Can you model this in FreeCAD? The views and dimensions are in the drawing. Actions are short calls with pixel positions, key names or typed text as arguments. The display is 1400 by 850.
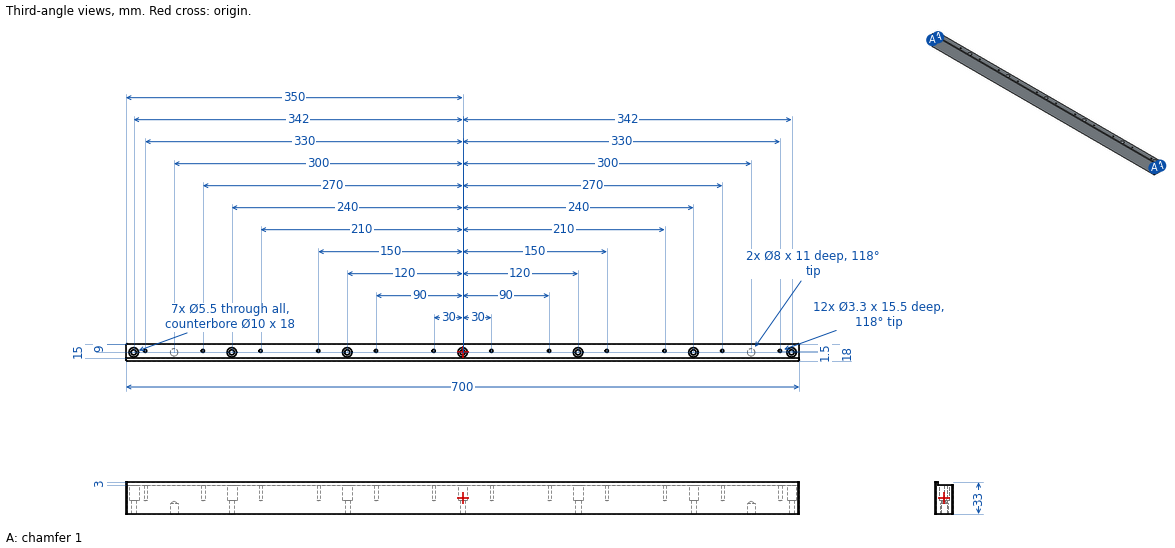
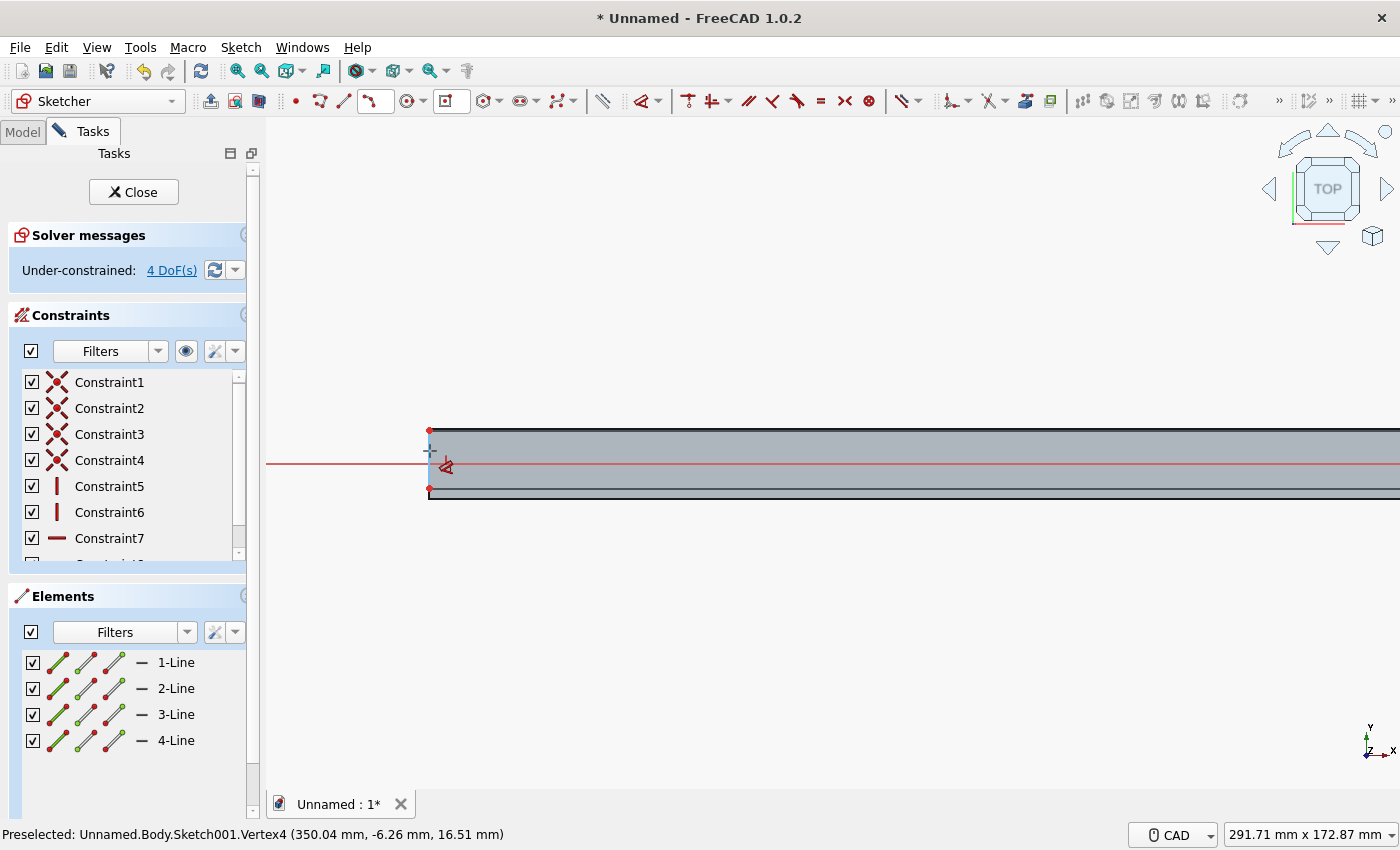
click(429, 448)
click(395, 446)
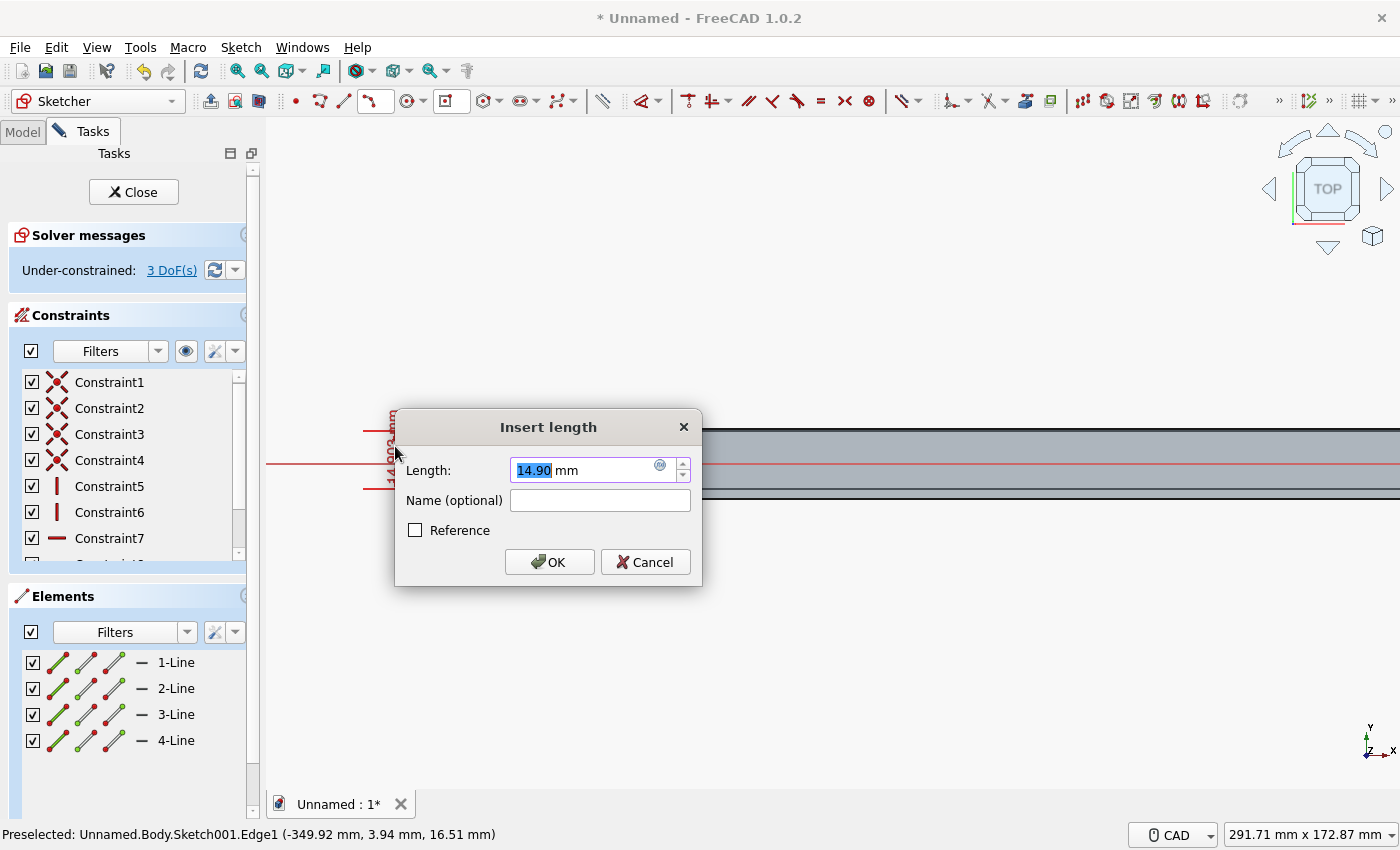
text(15)
key(Return)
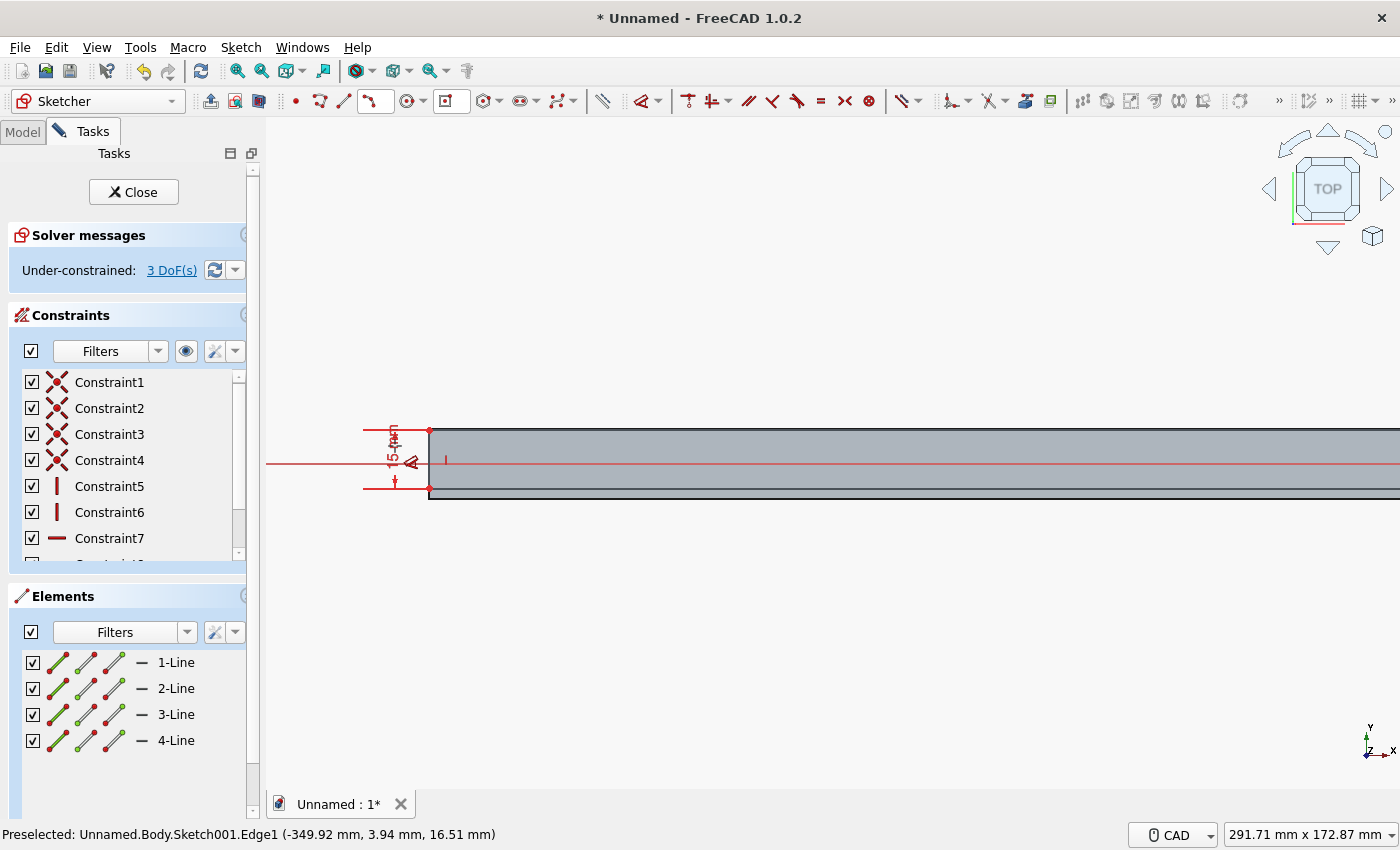
click(429, 430)
click(323, 447)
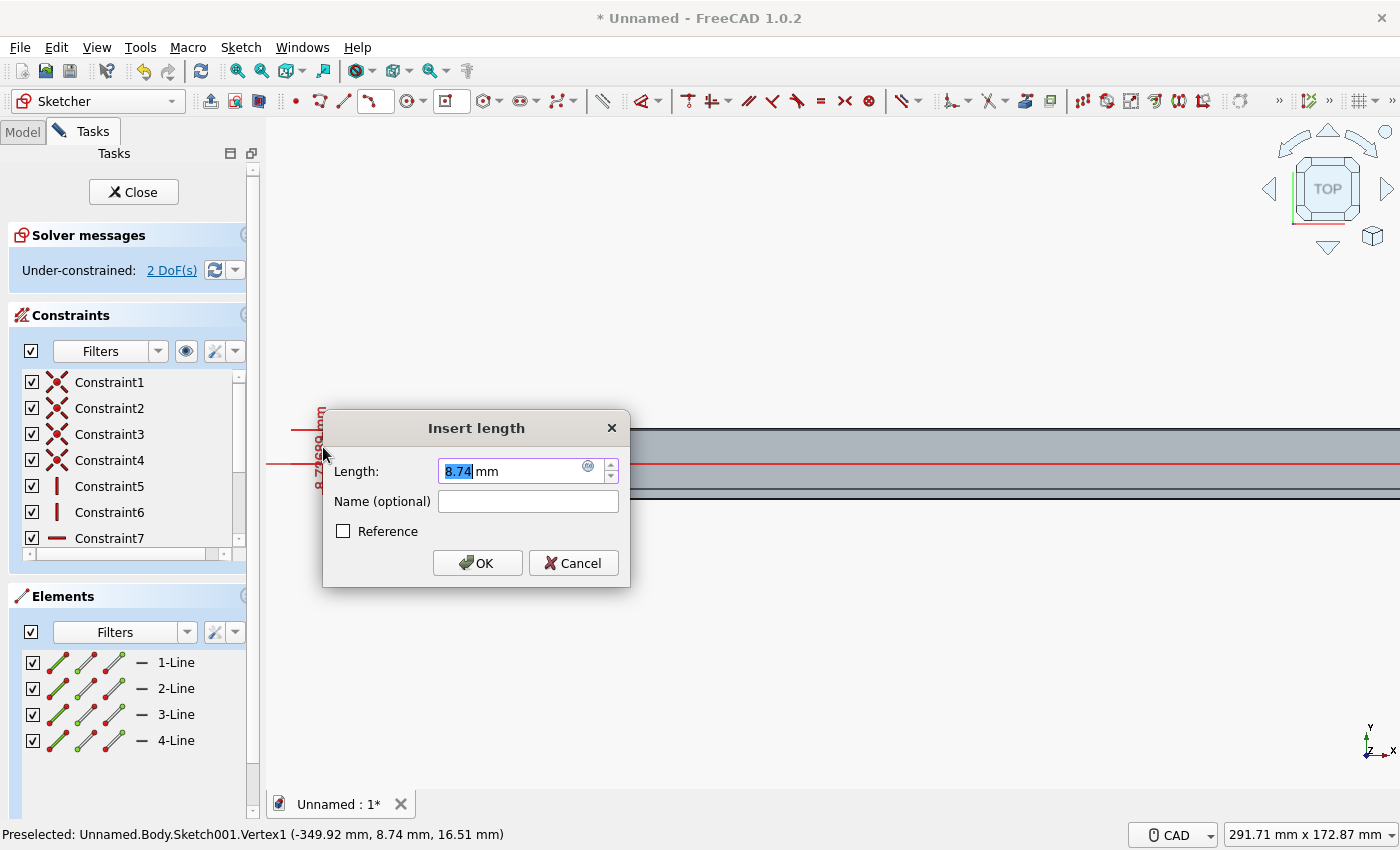
text(9)
key(Return)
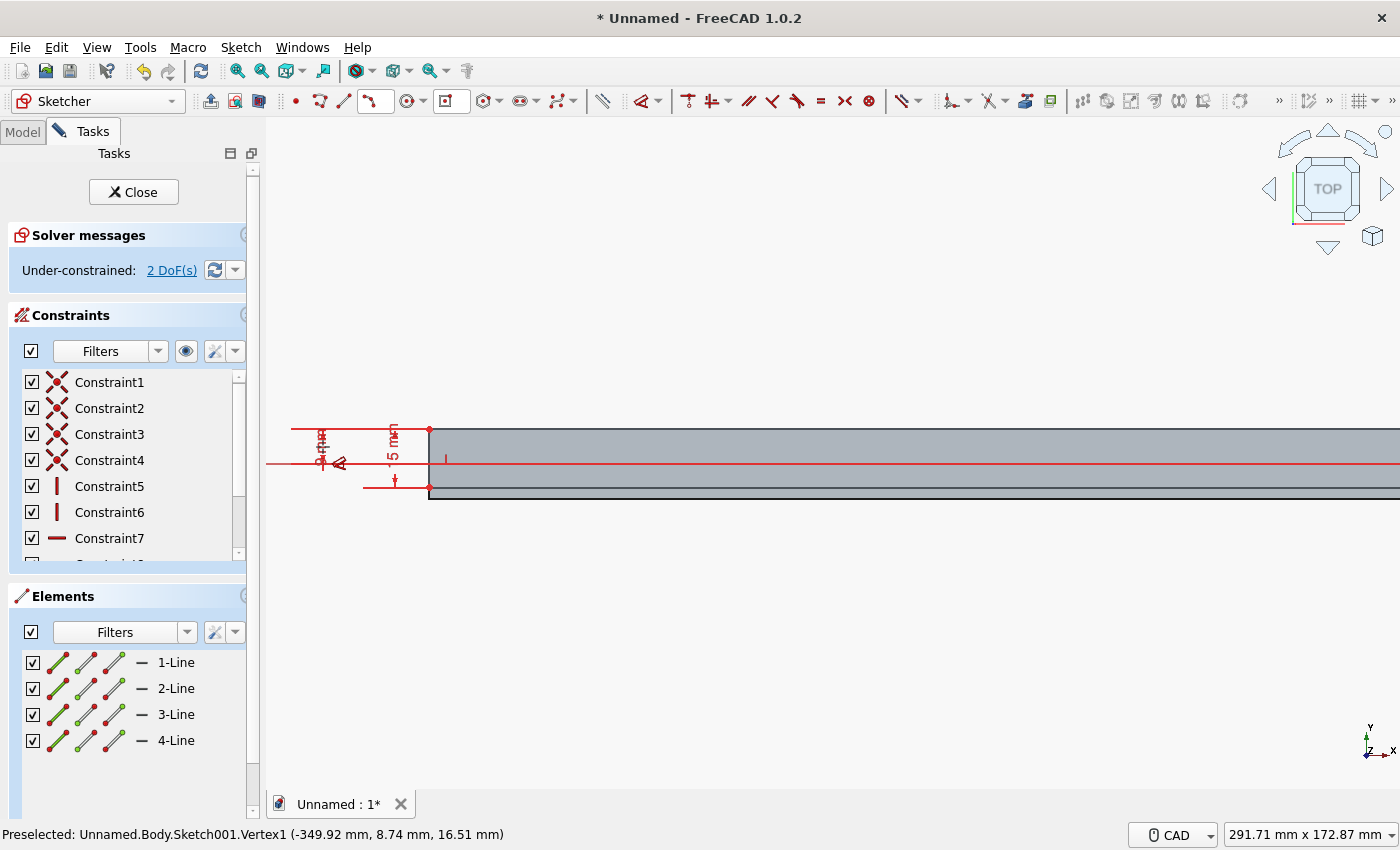
click(973, 488)
click(832, 522)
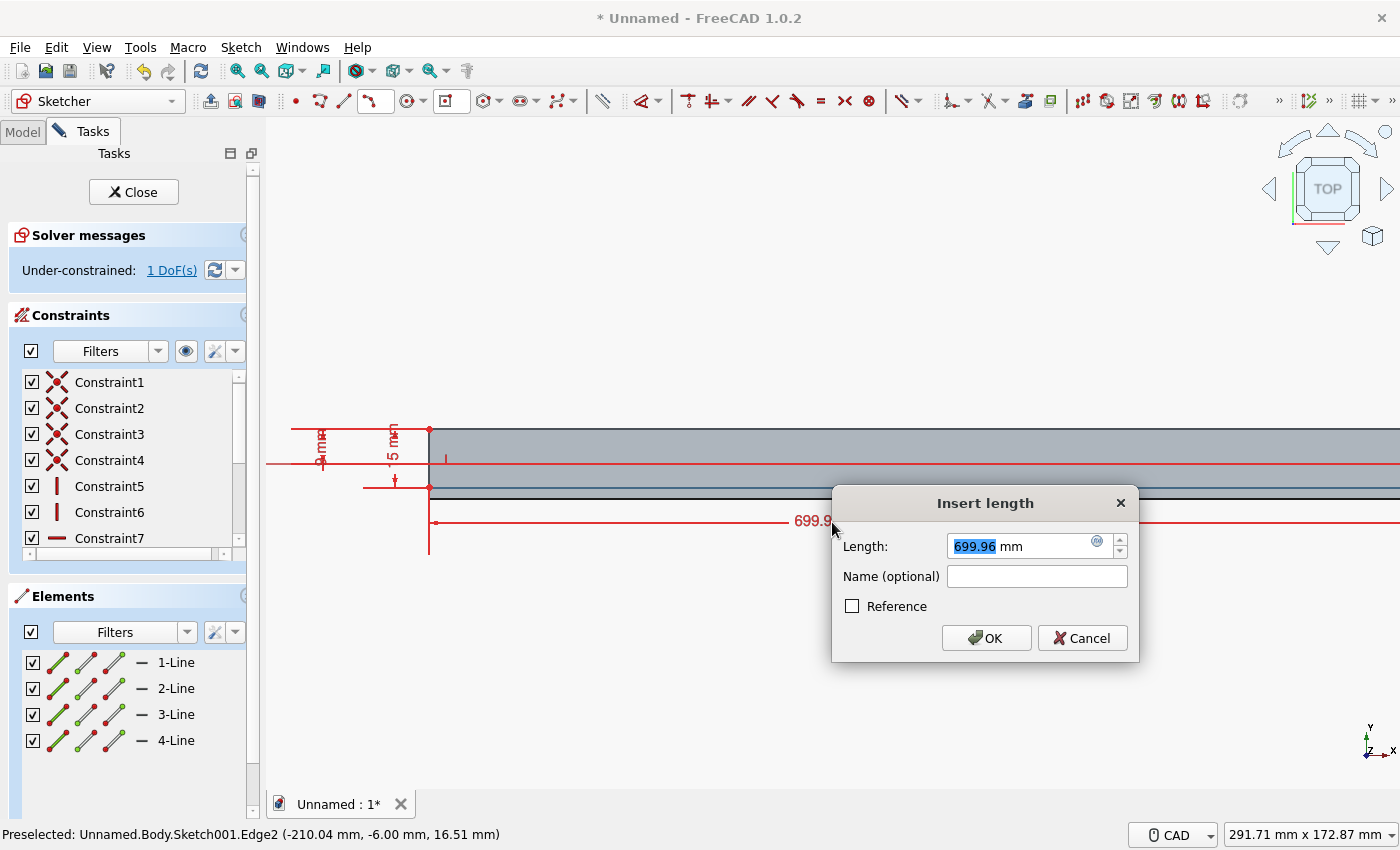
text(700)
key(Return)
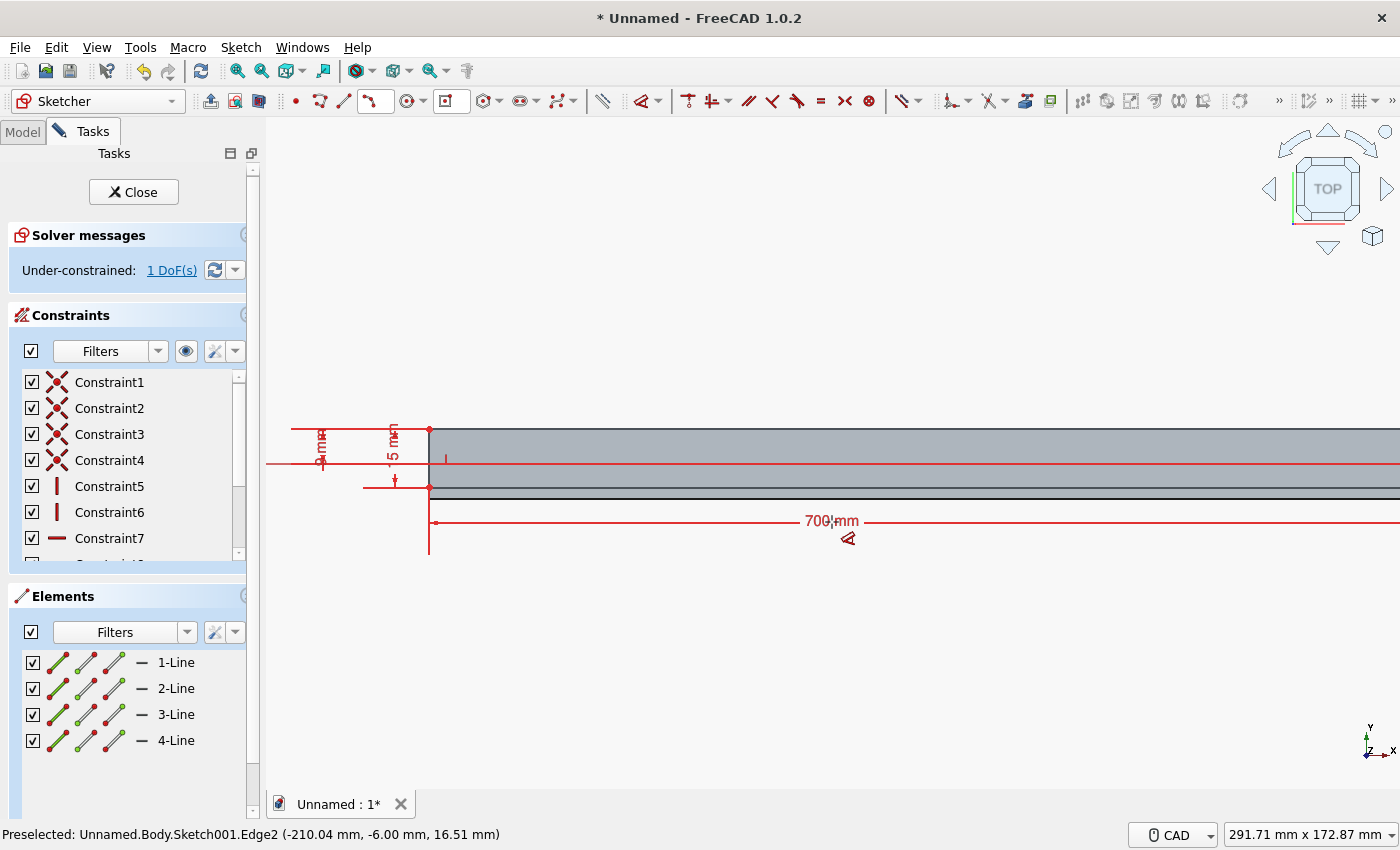
scroll(429, 451, down, 7)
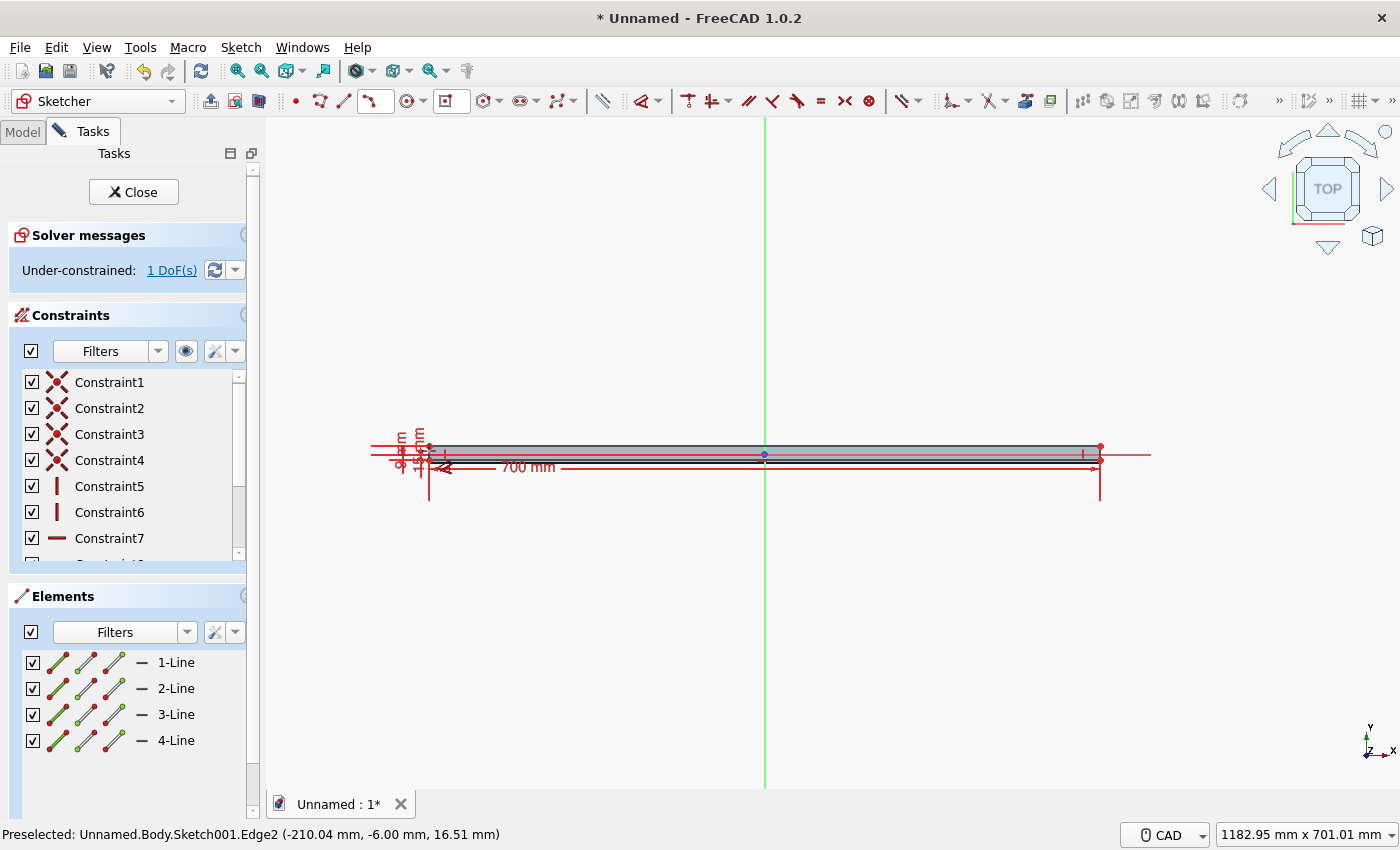
click(429, 446)
click(597, 412)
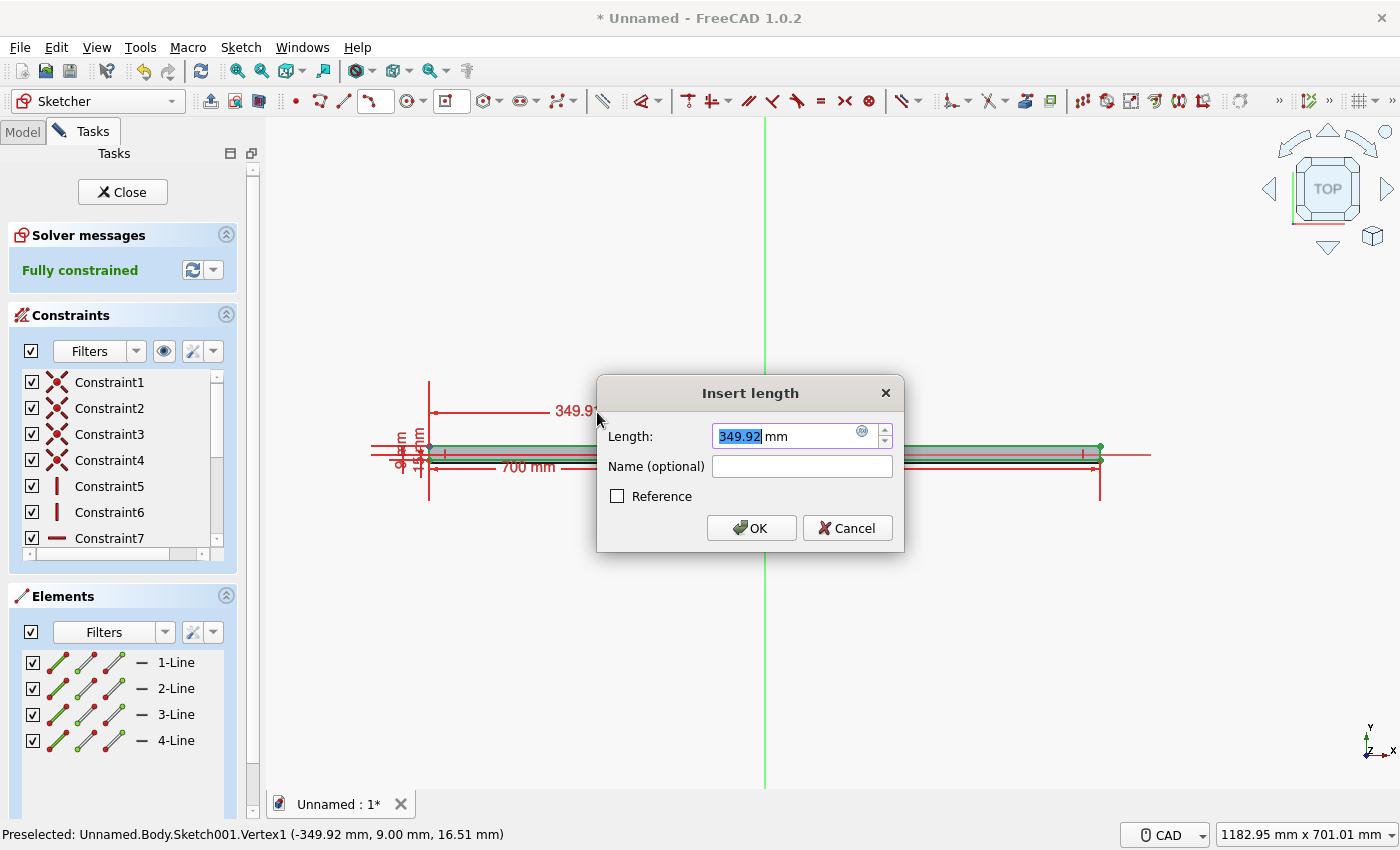
text(350)
key(Return)
key(Escape)